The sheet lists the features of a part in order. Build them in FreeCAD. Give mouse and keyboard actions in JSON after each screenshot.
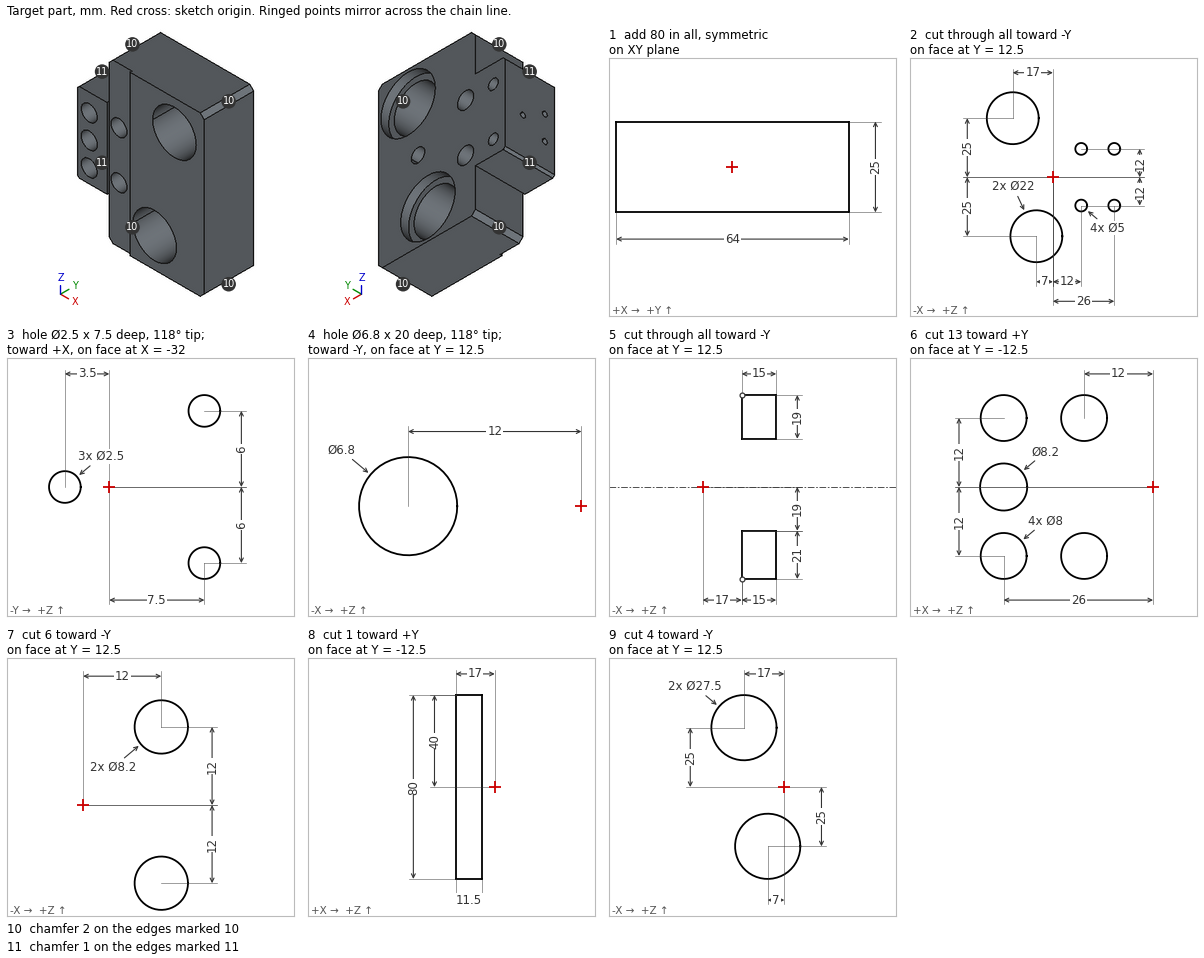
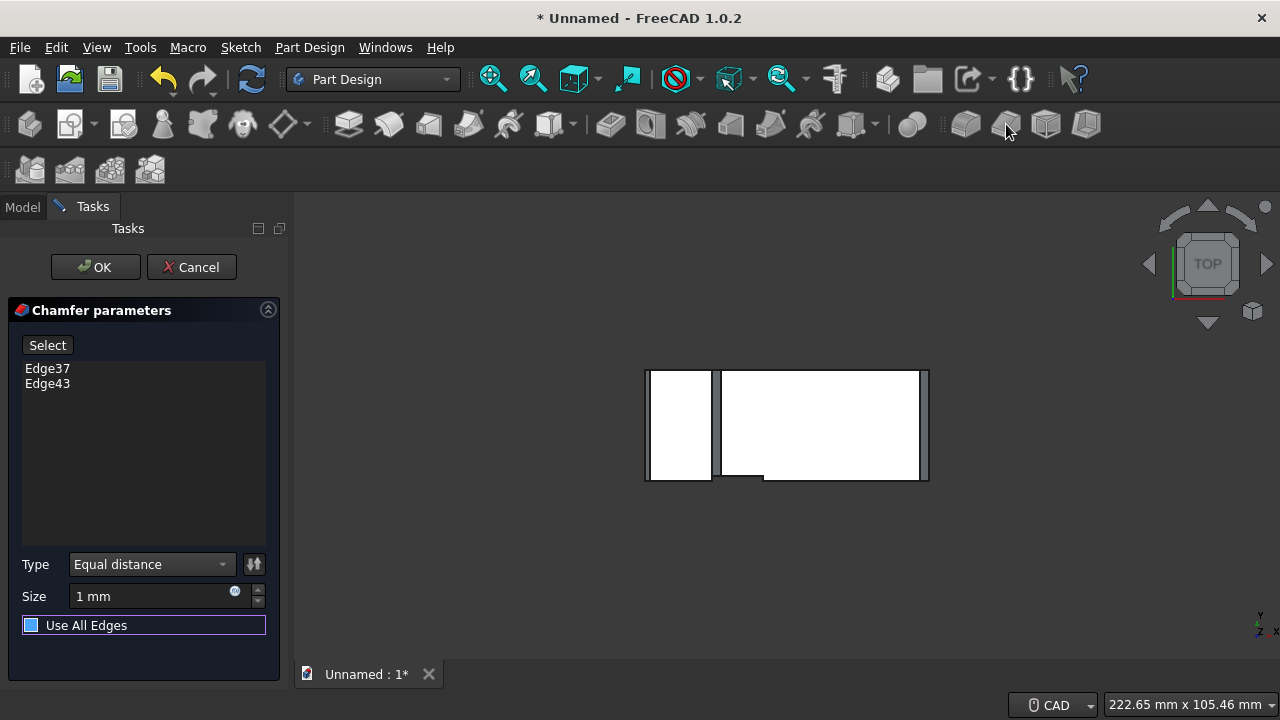
{"action": "left_click", "coordinate": [96, 267]}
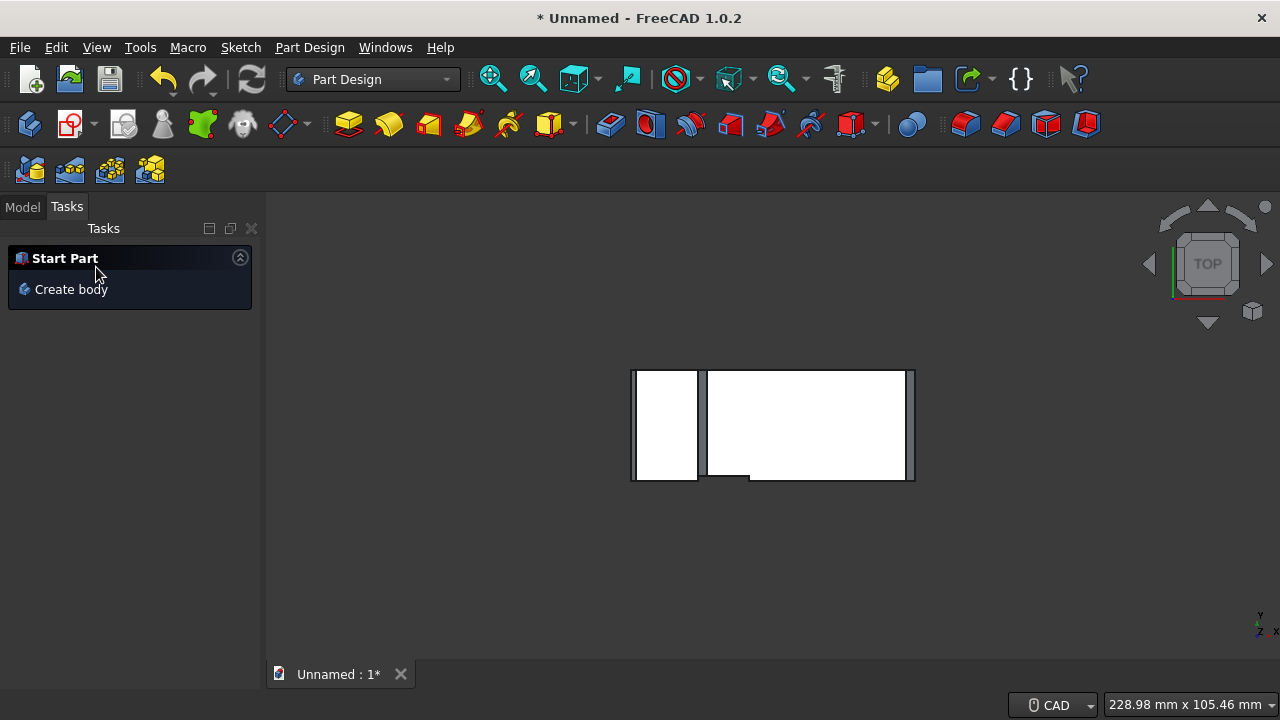
{"action": "key", "text": "0"}